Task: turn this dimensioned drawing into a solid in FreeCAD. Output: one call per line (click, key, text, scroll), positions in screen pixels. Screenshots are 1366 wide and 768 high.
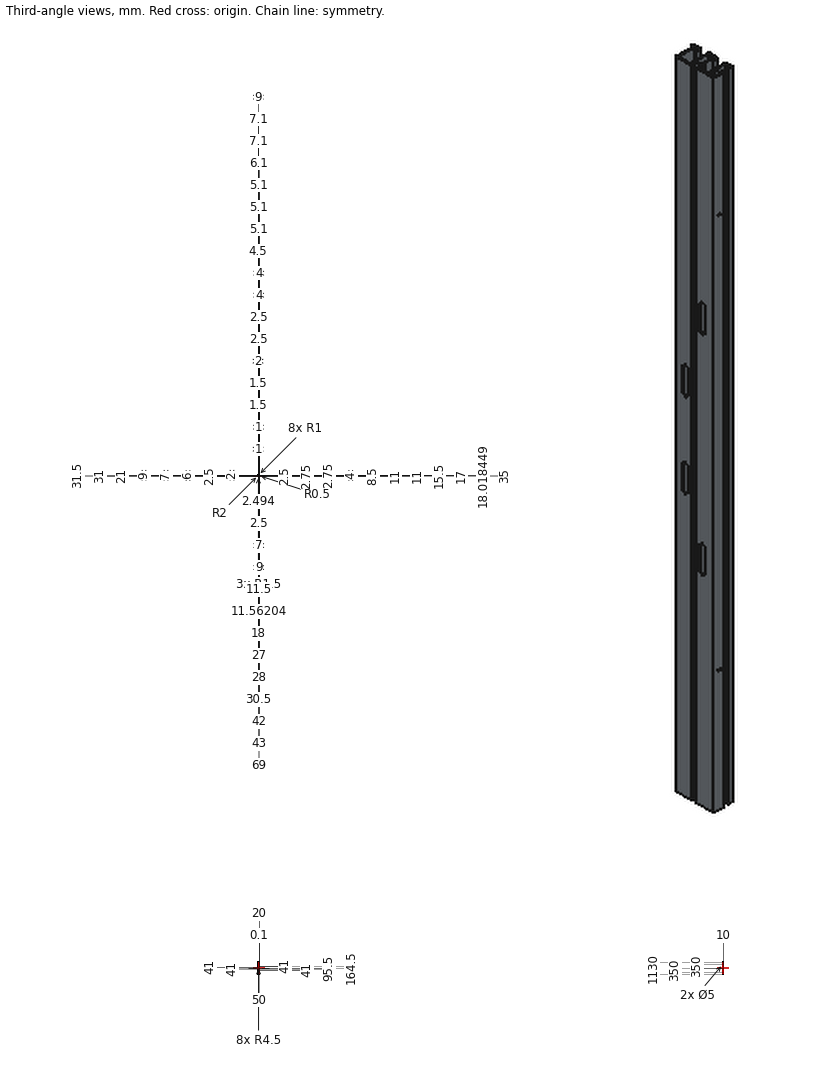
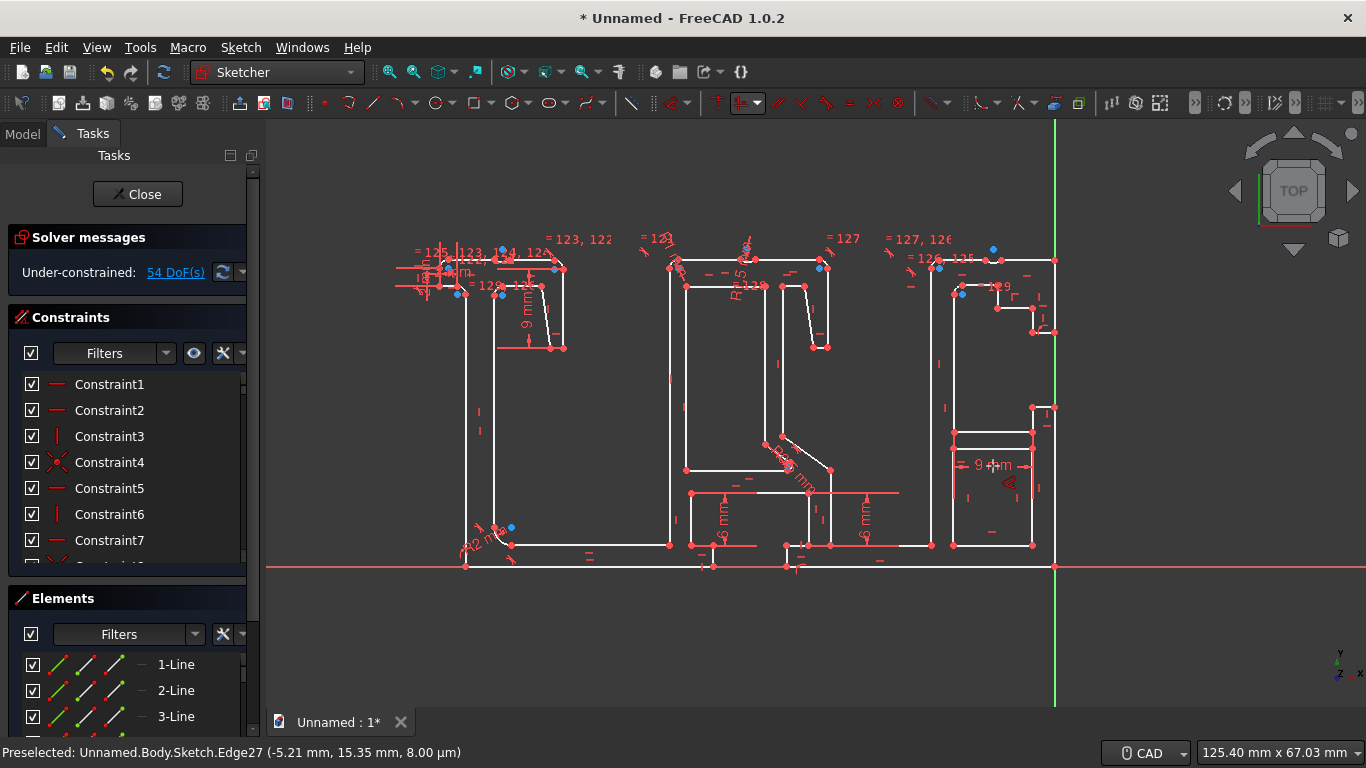
scroll(973, 285, up, 2)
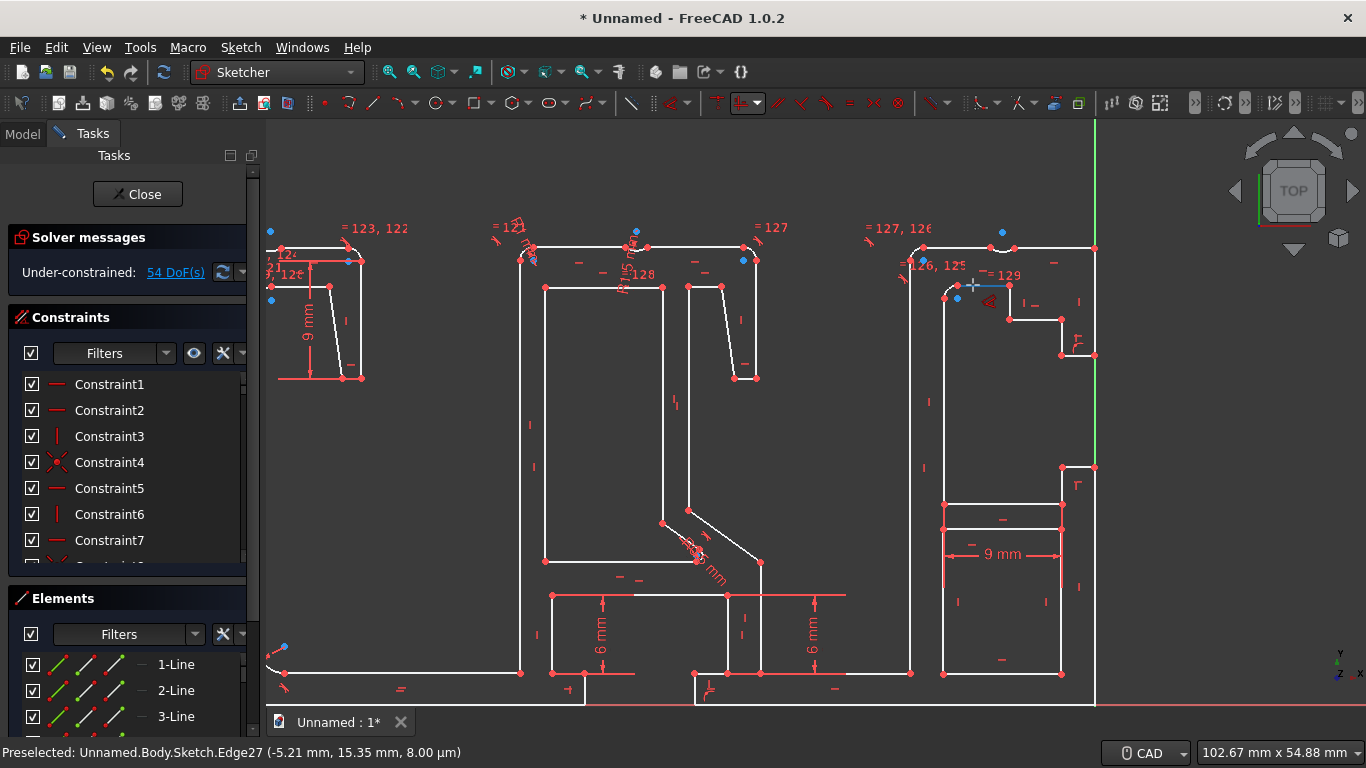
click(973, 286)
click(984, 320)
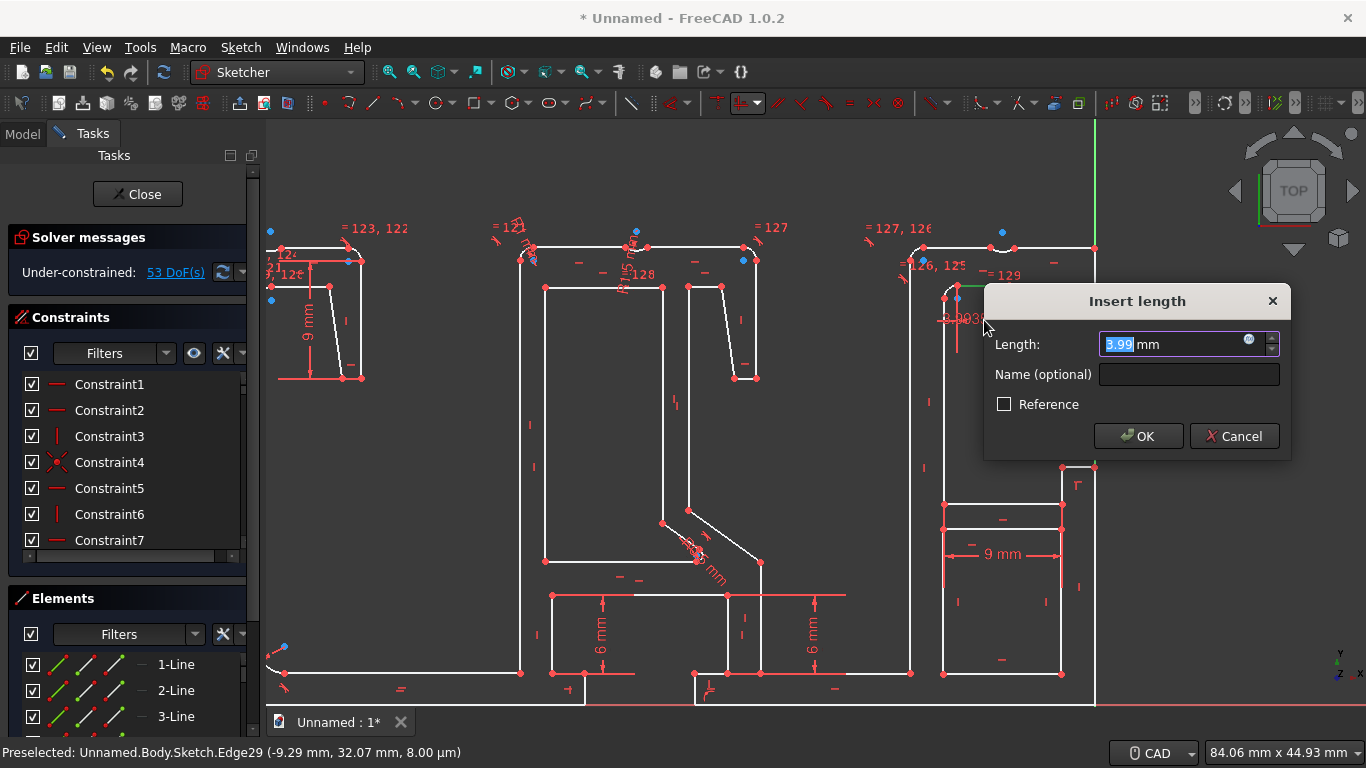
text(4)
key(Return)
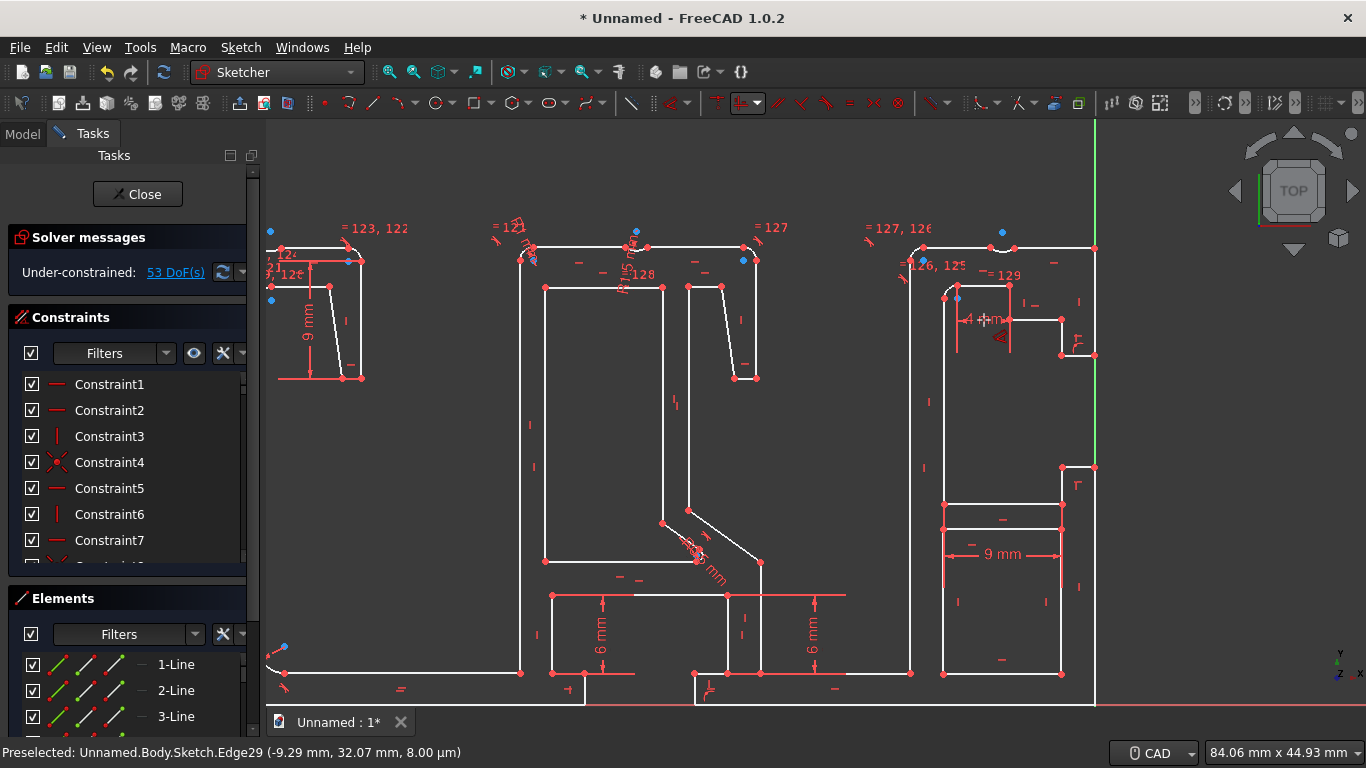
click(1025, 320)
click(1036, 286)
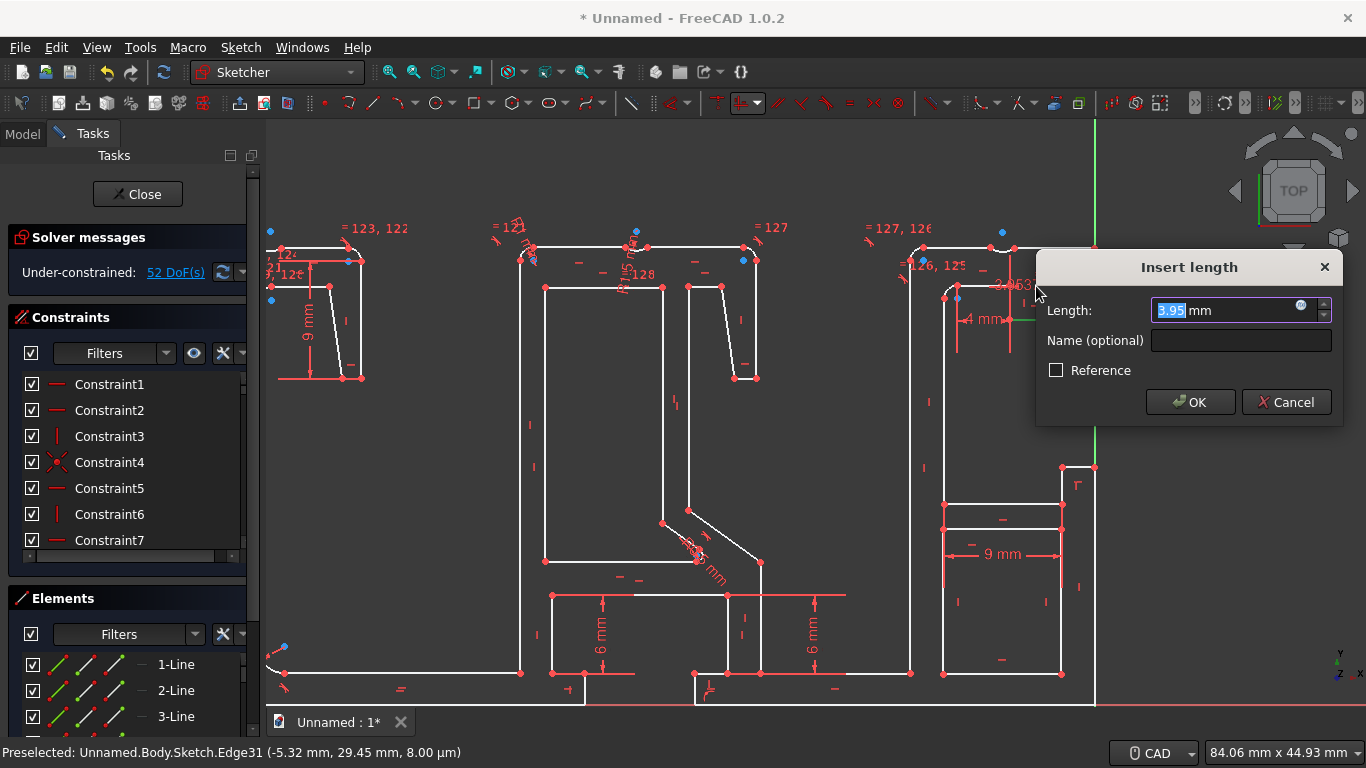
text(4)
key(Return)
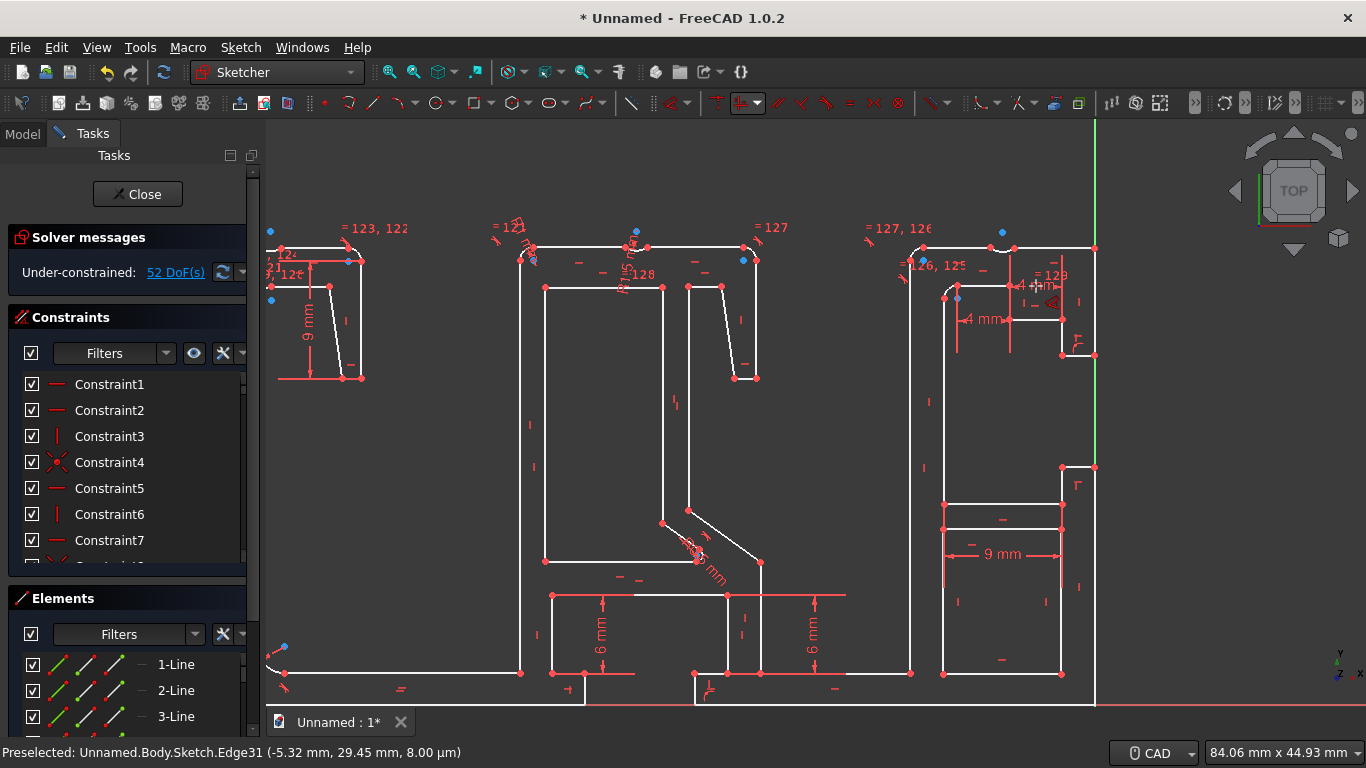
click(756, 343)
click(790, 319)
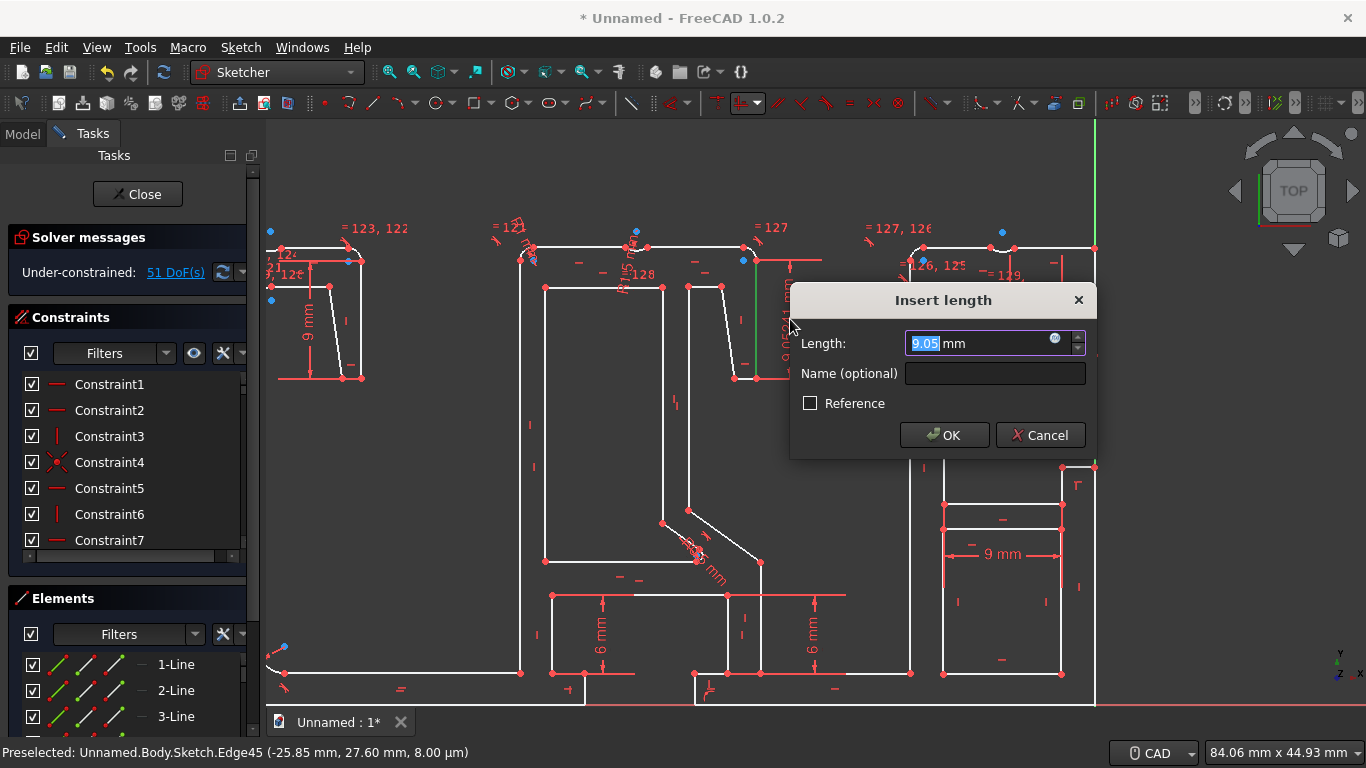
text(9)
key(Return)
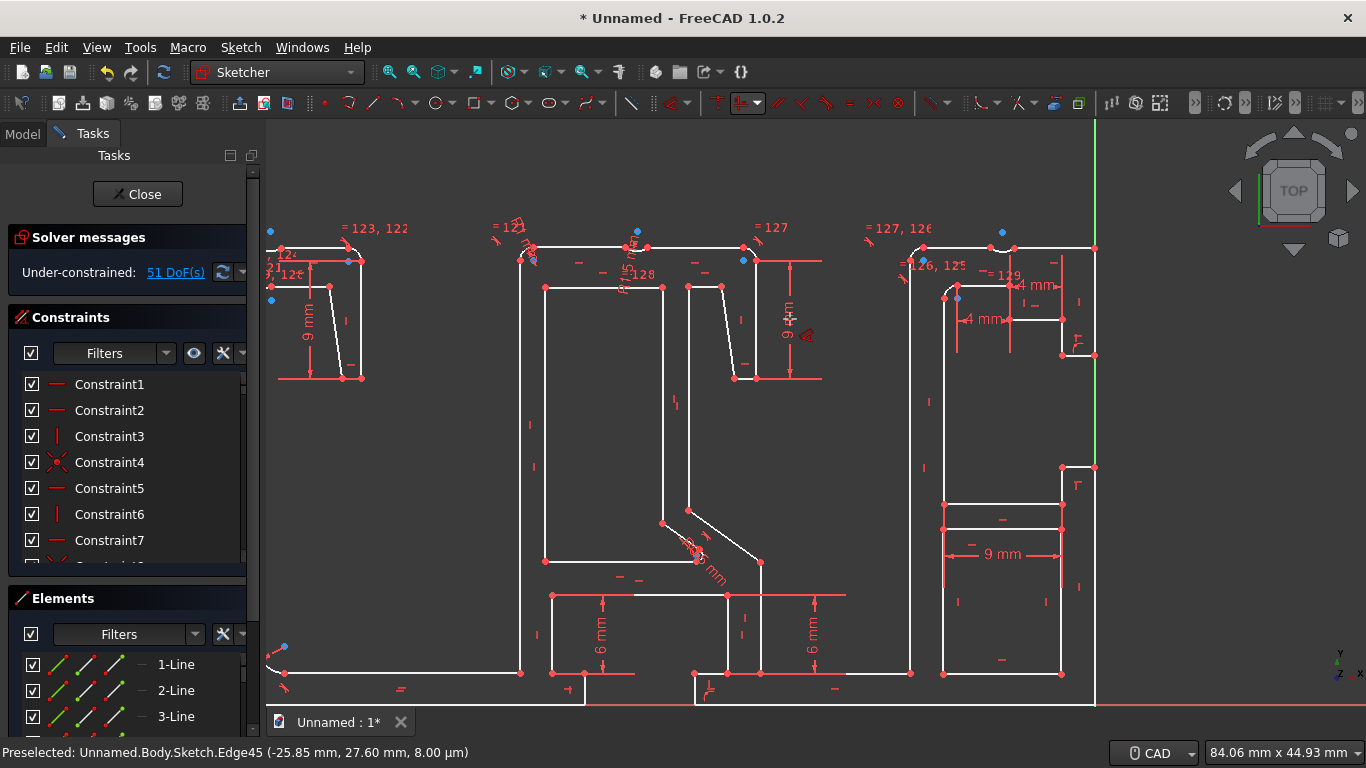
click(979, 674)
click(1002, 640)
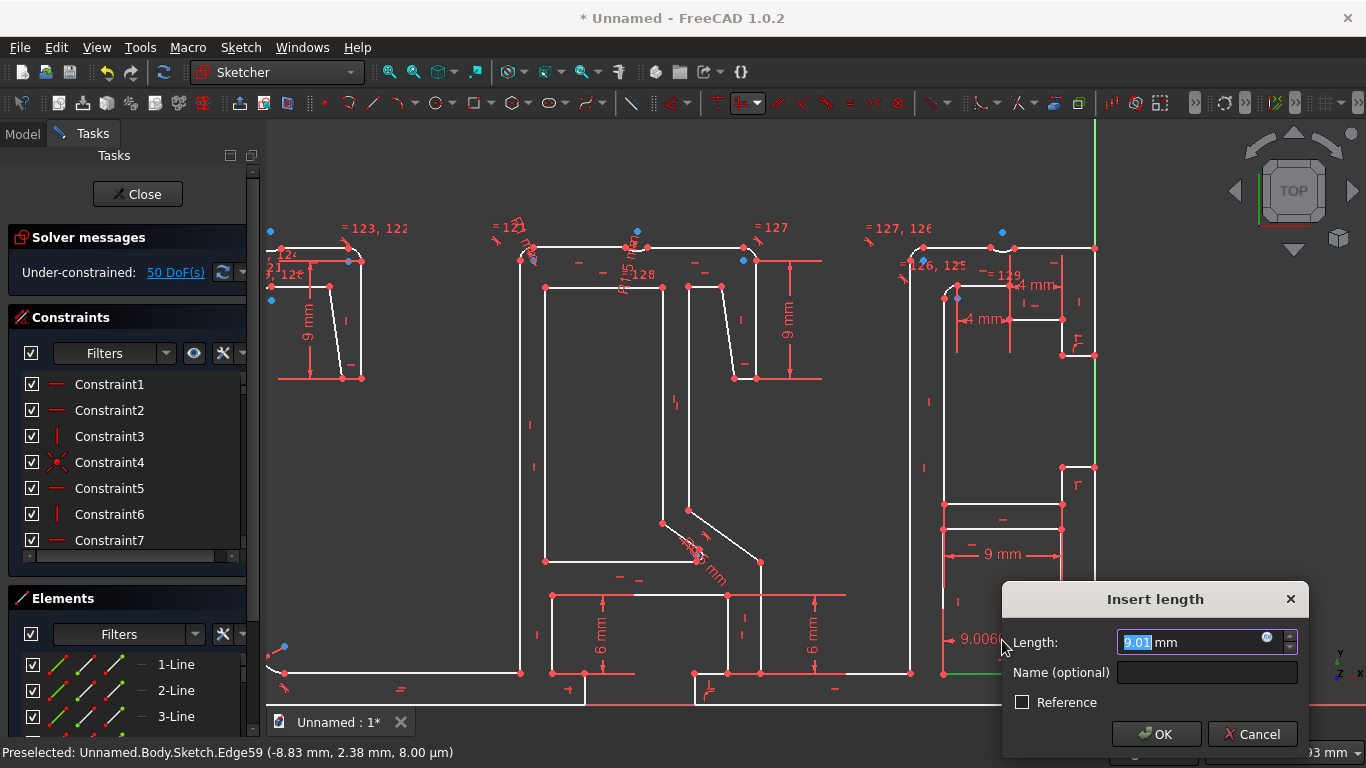
text(9)
key(Return)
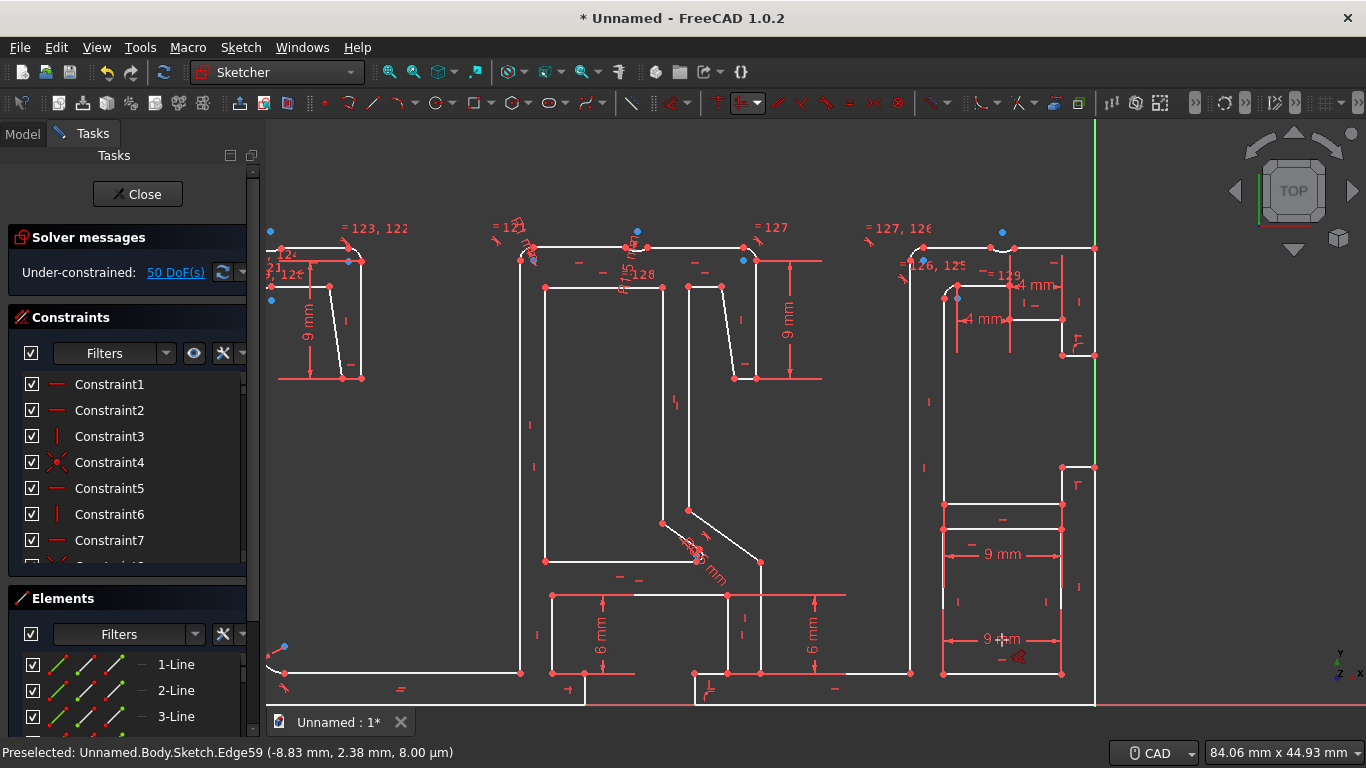
click(580, 288)
click(604, 322)